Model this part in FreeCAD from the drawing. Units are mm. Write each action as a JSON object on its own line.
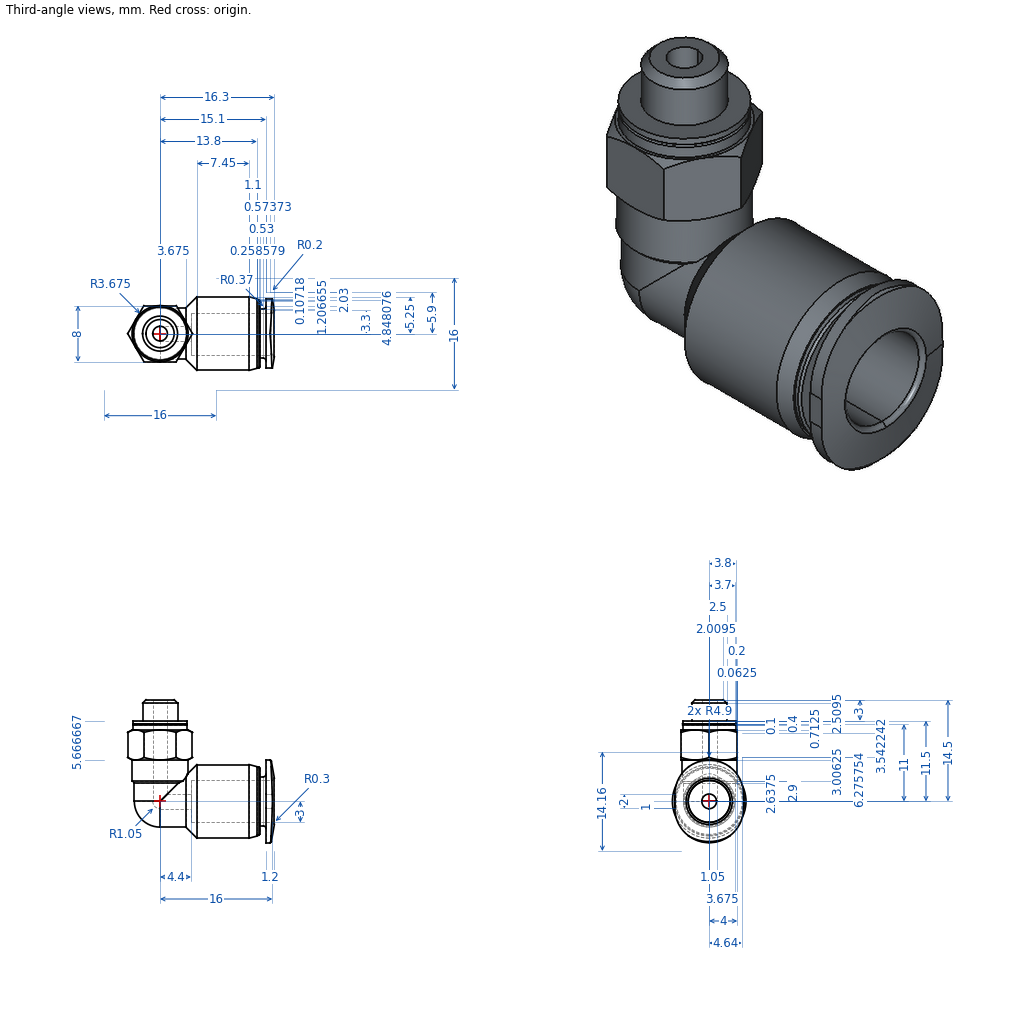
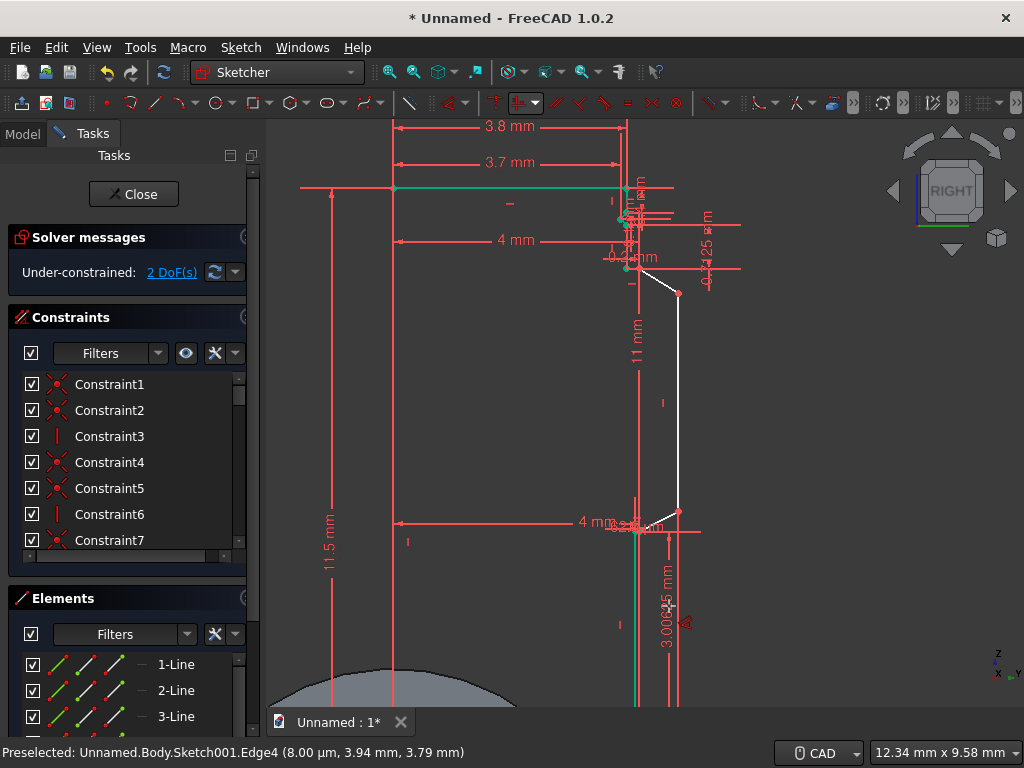
{"action": "left_click", "coordinate": [678, 446]}
{"action": "left_click", "coordinate": [712, 402]}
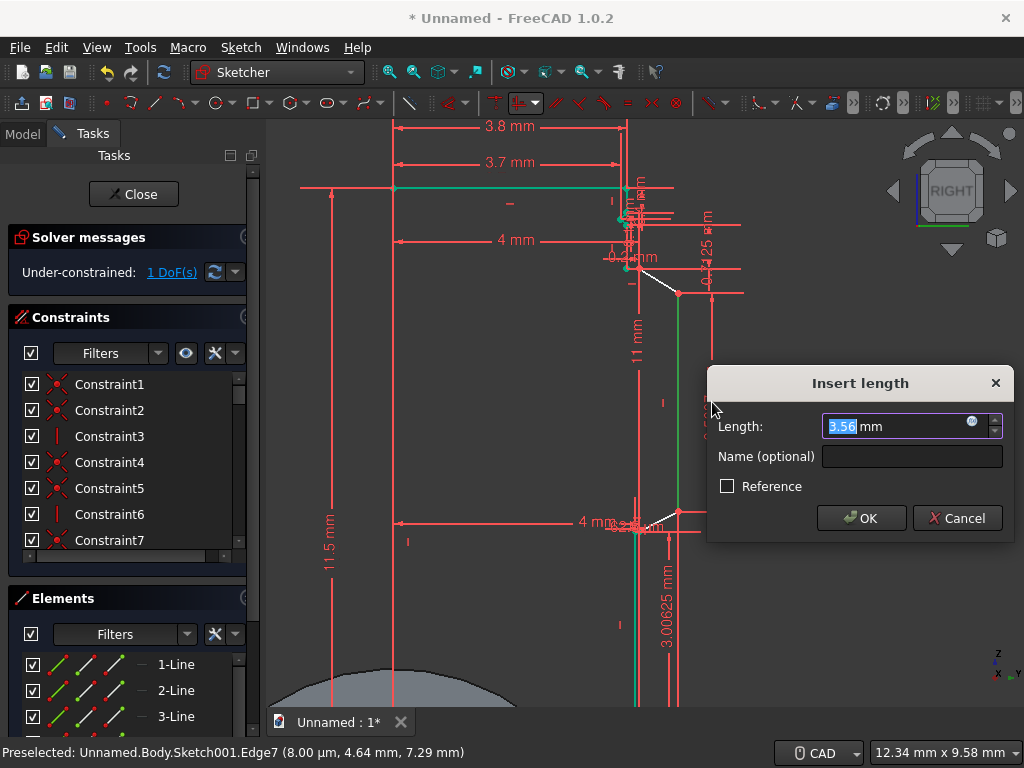
{"action": "type", "text": "3.542242"}
{"action": "key", "text": "Return"}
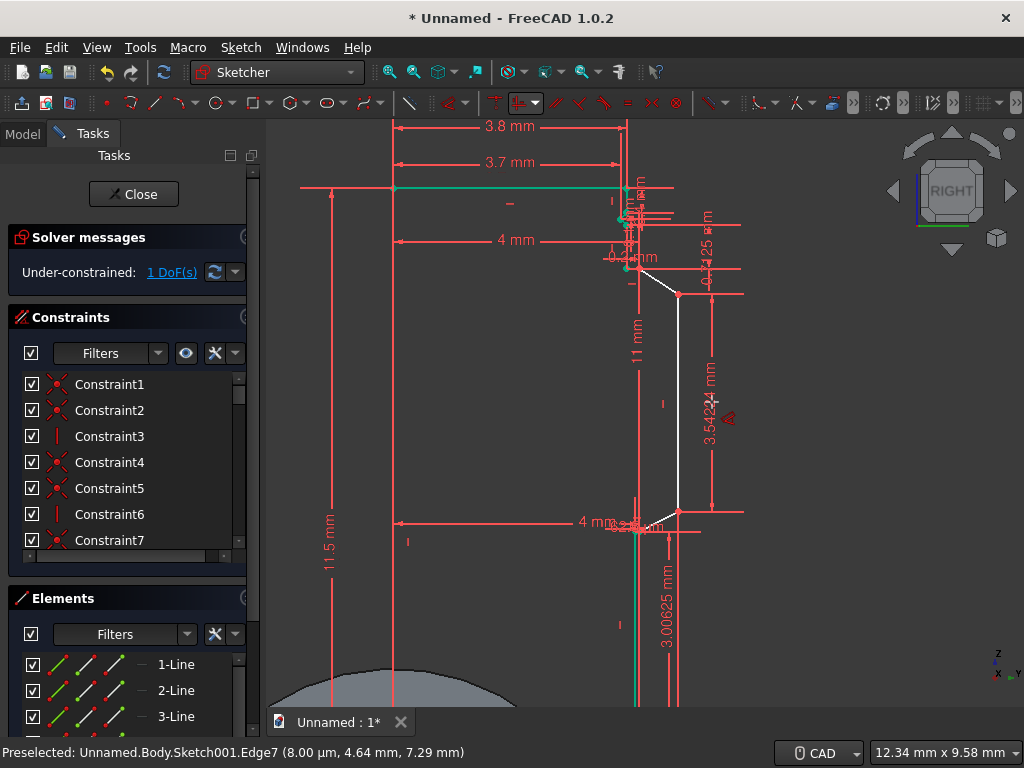
{"action": "left_click", "coordinate": [678, 512]}
{"action": "left_click", "coordinate": [712, 557]}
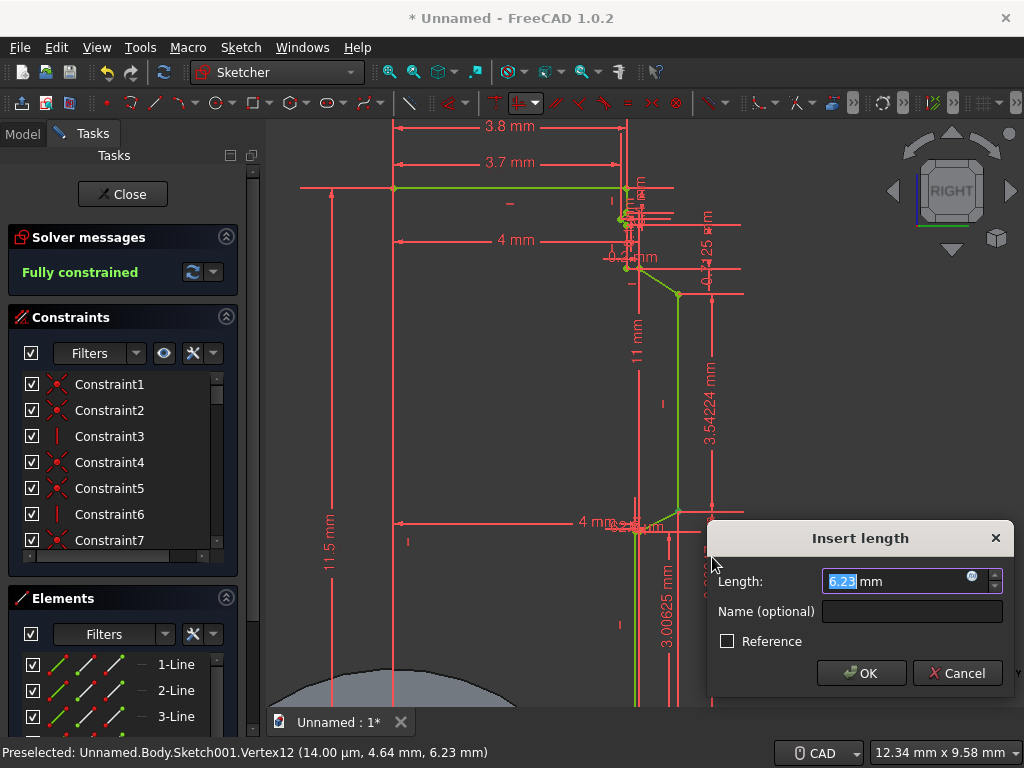
{"action": "type", "text": "6.275754"}
{"action": "key", "text": "Return"}
{"action": "key", "text": "Escape"}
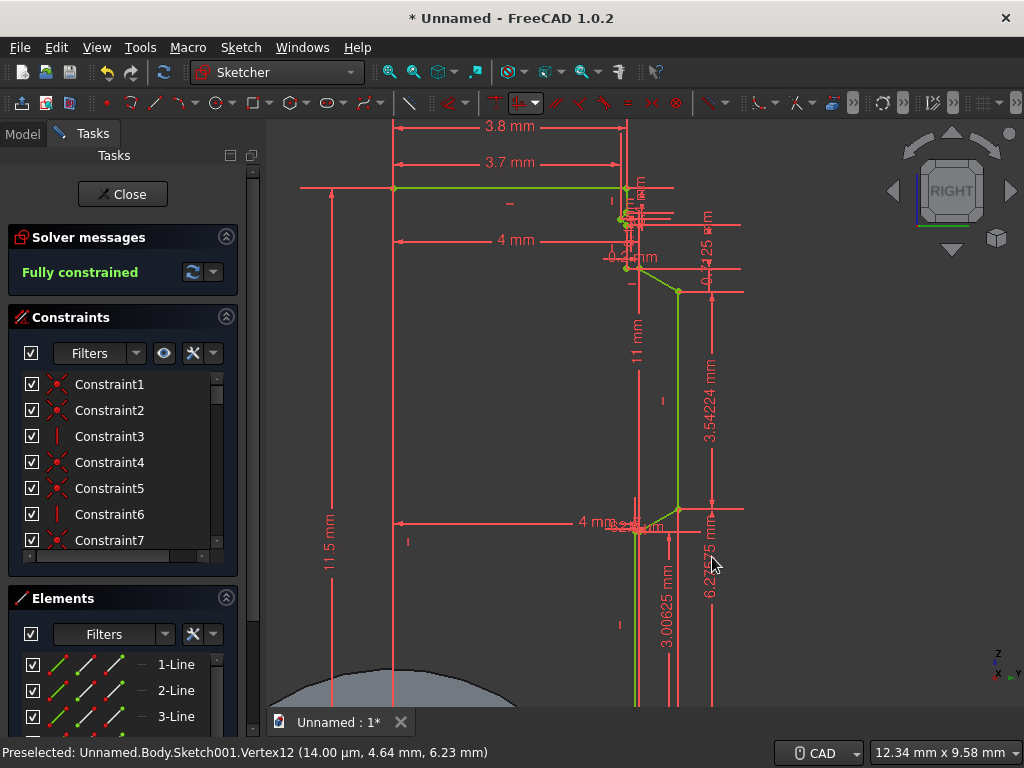
{"action": "left_click", "coordinate": [123, 194]}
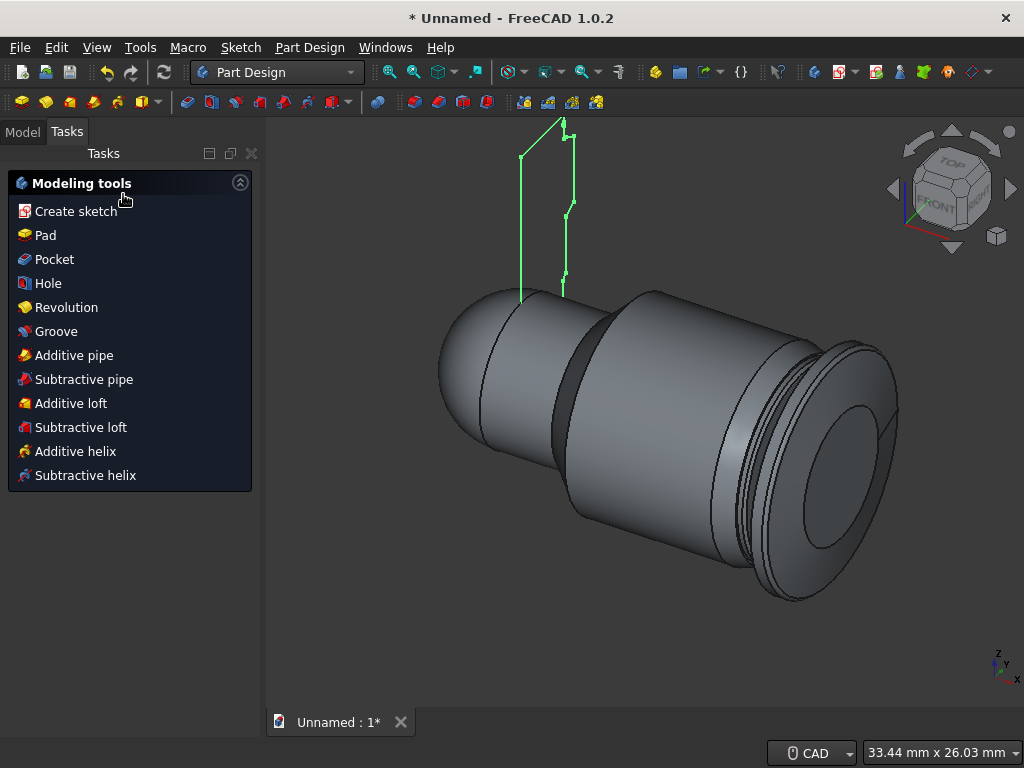
{"action": "left_click", "coordinate": [46, 102]}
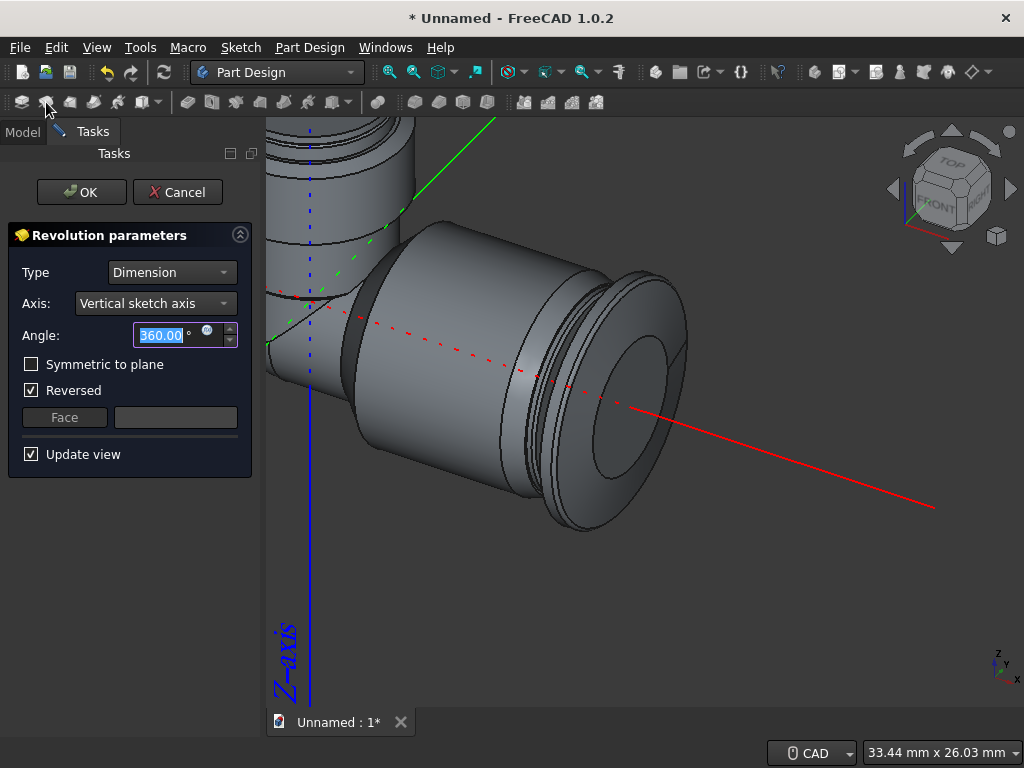
{"action": "left_click", "coordinate": [82, 192]}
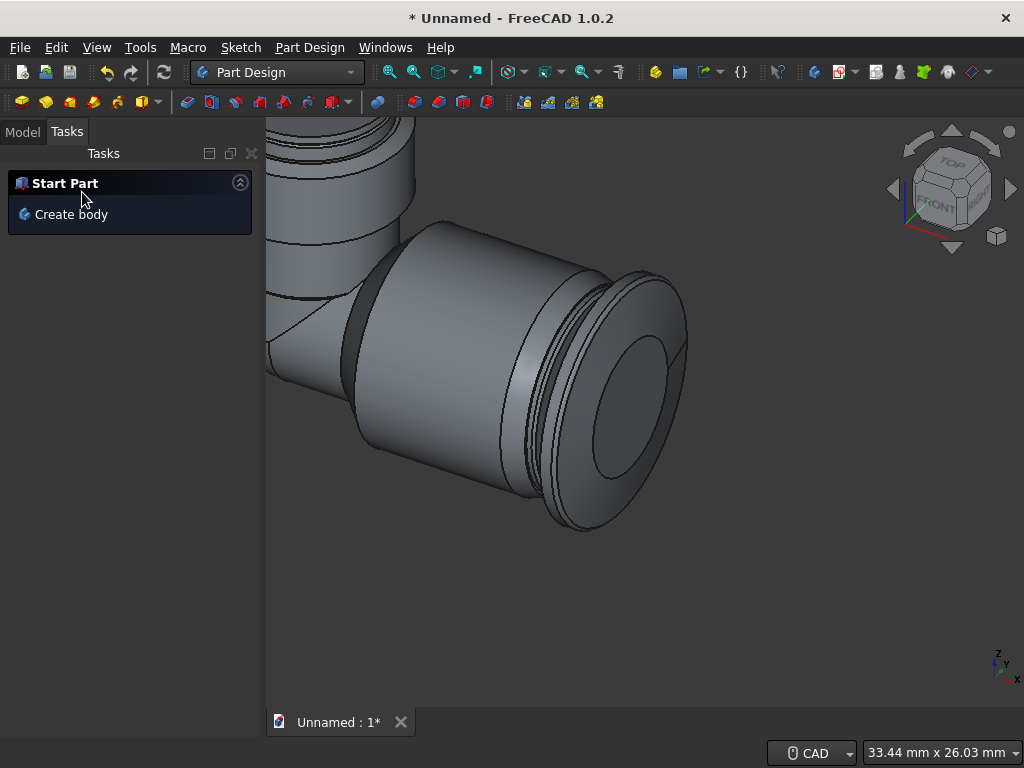
{"action": "left_click", "coordinate": [390, 72]}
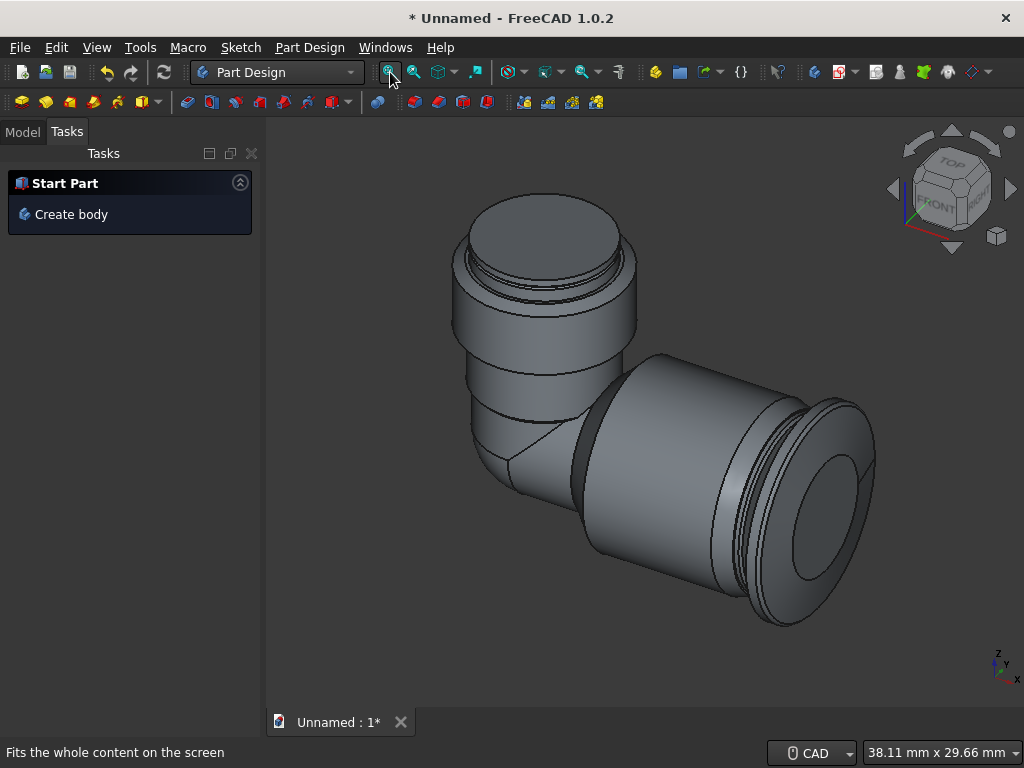
{"action": "left_click", "coordinate": [840, 72]}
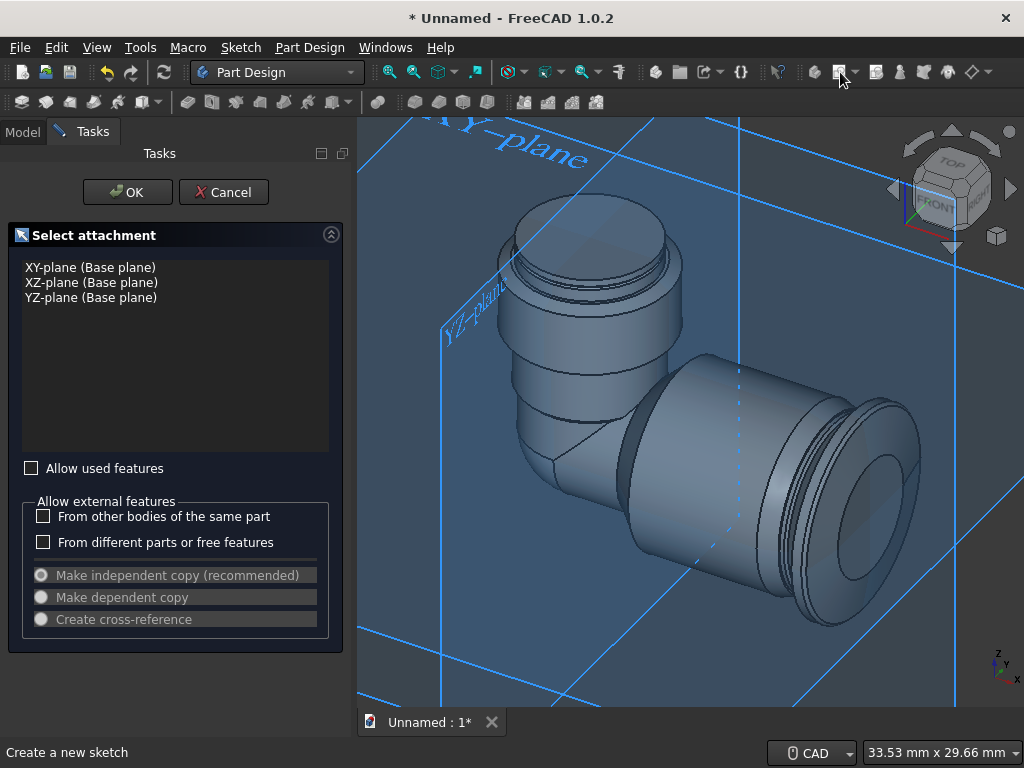
{"action": "left_click", "coordinate": [82, 298]}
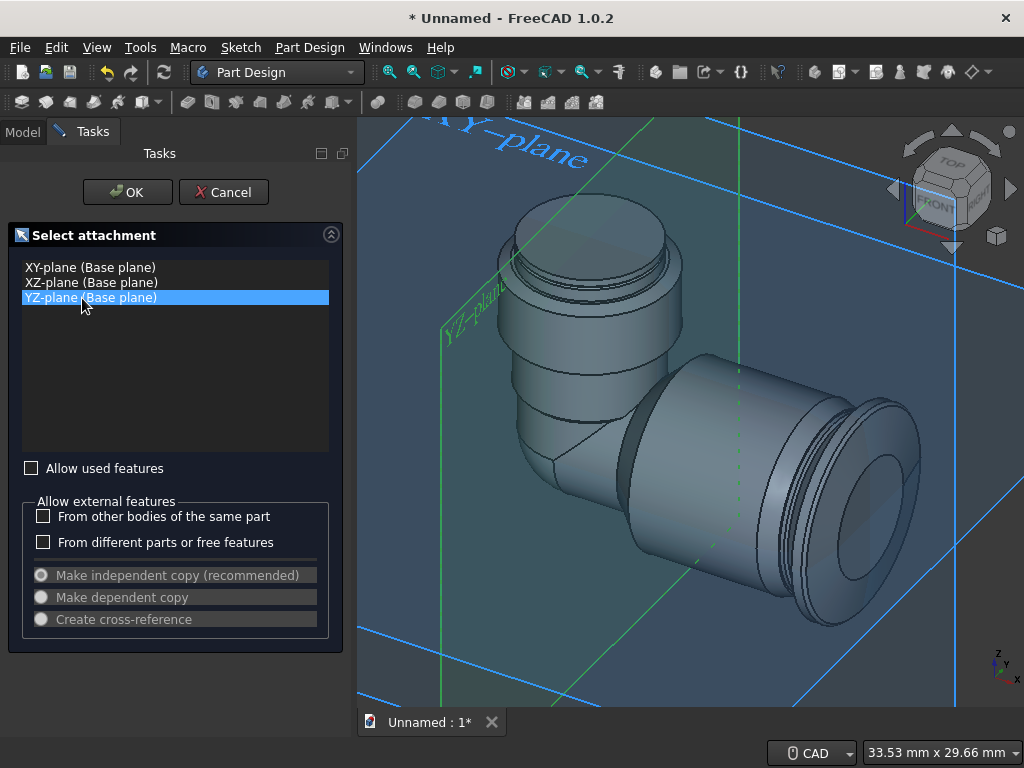
{"action": "left_click", "coordinate": [128, 192]}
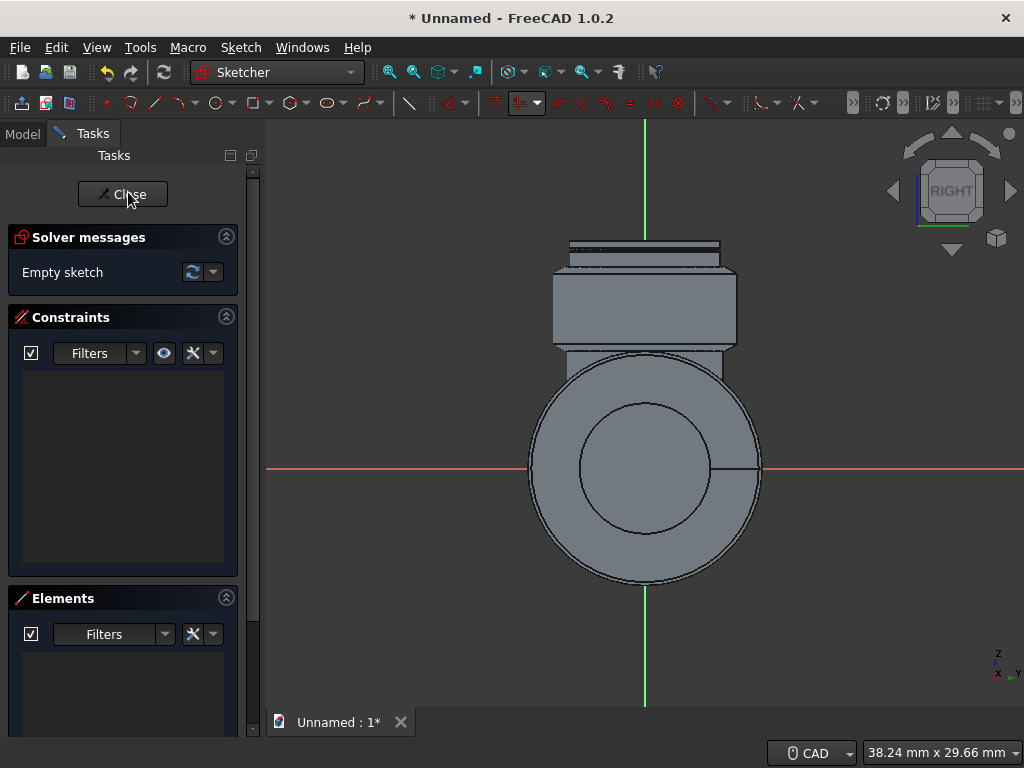
{"action": "left_click", "coordinate": [70, 104]}